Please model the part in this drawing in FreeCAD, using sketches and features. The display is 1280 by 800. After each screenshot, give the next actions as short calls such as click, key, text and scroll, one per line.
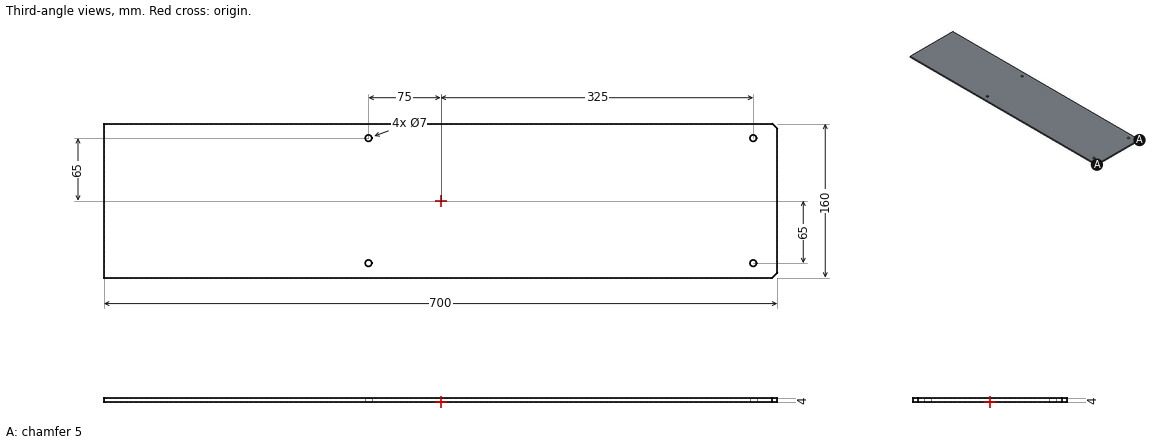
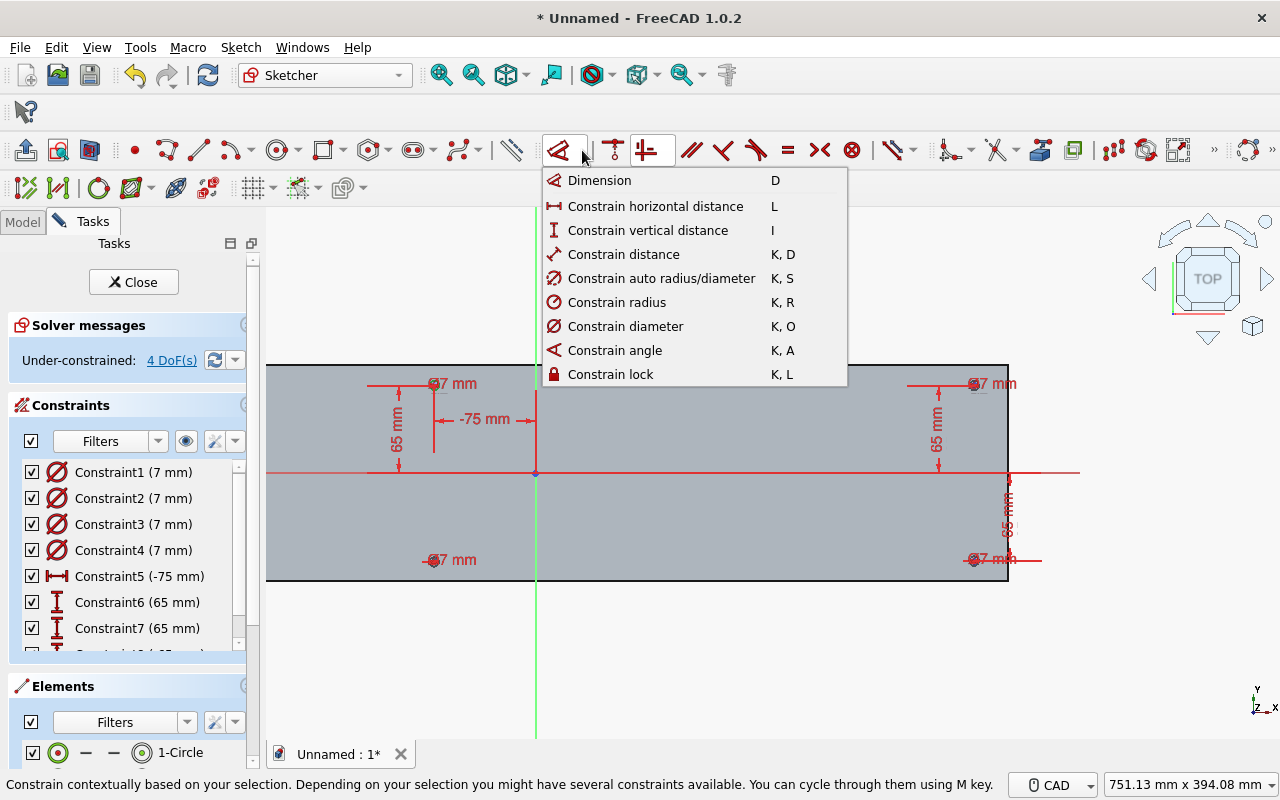
click(695, 206)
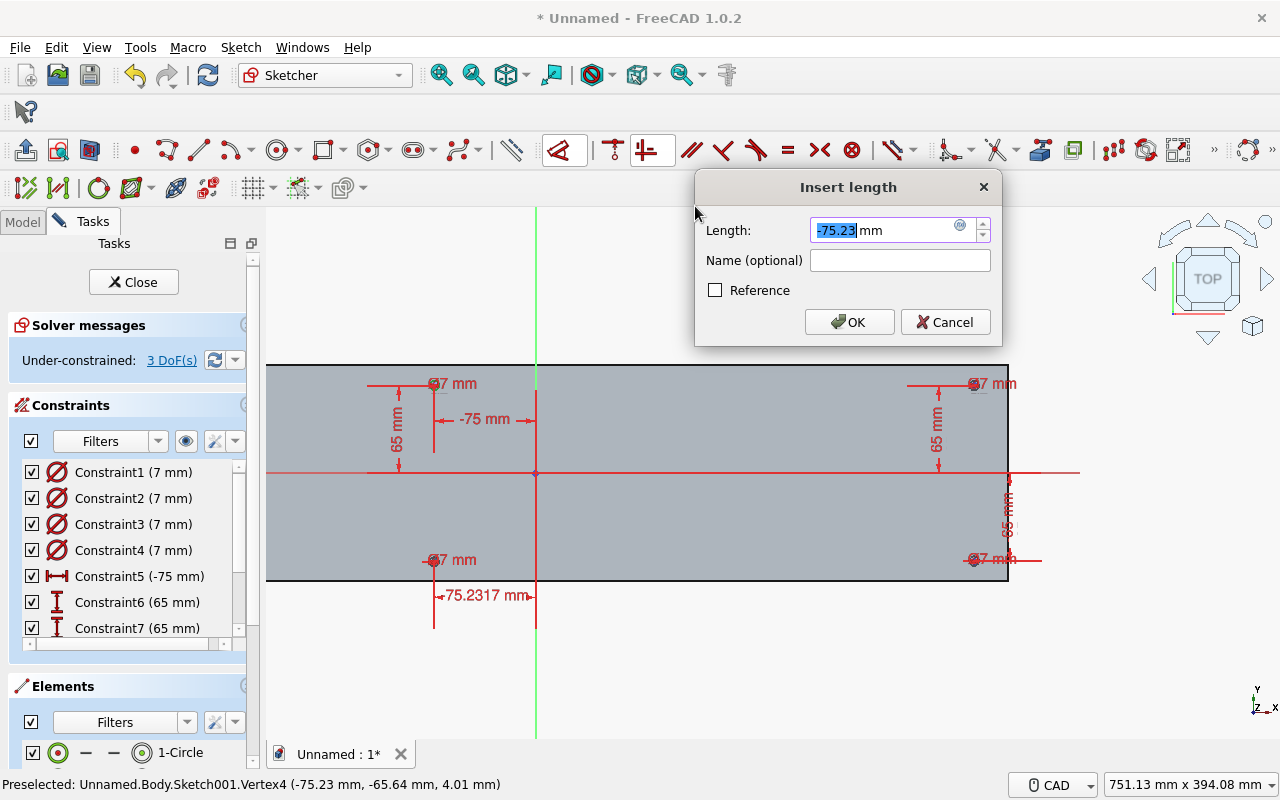
text(-75)
key(Return)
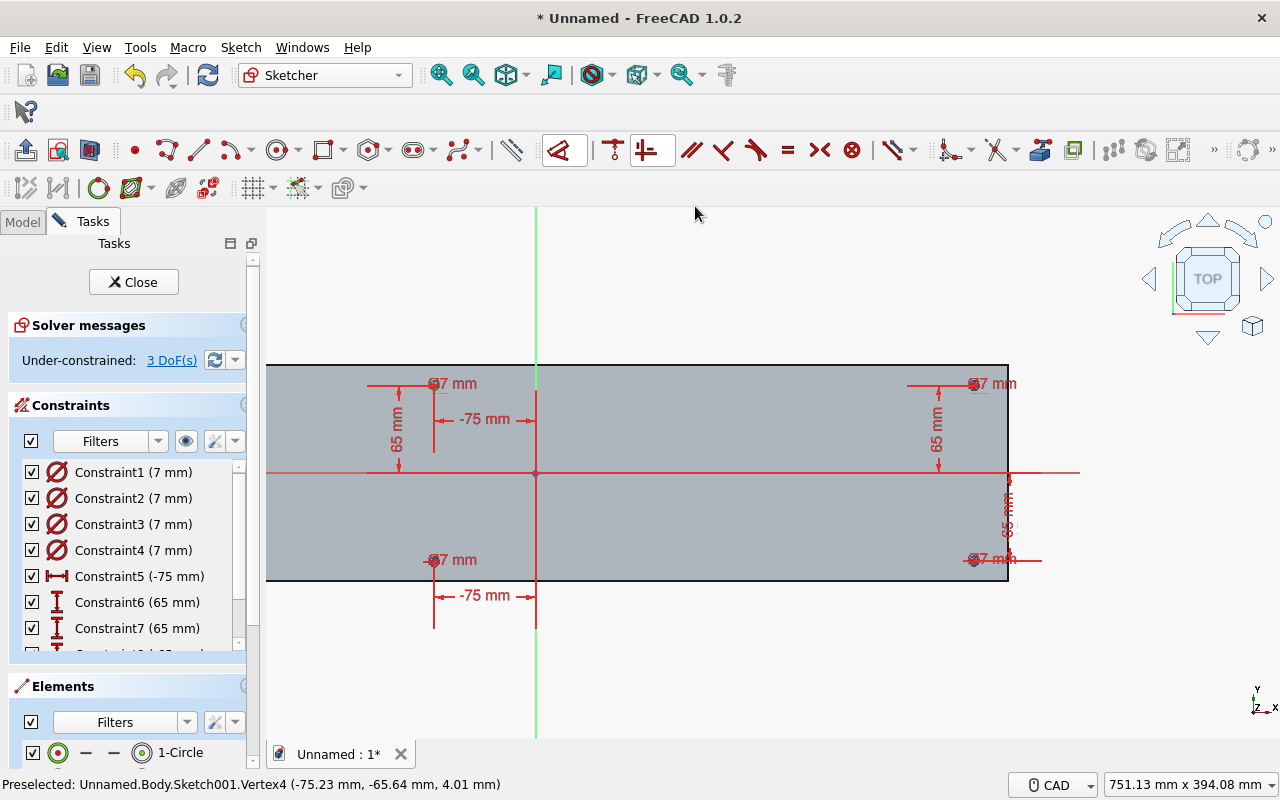
click(434, 562)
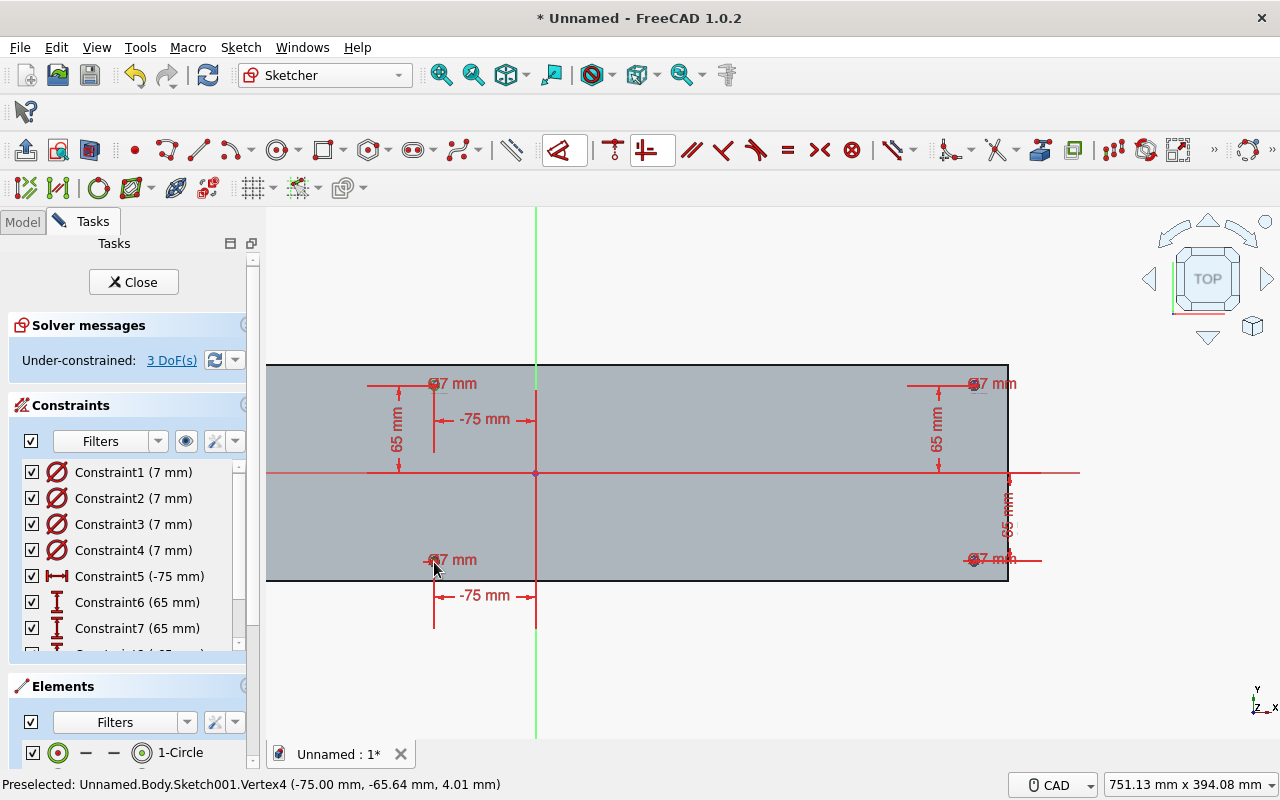
key(i)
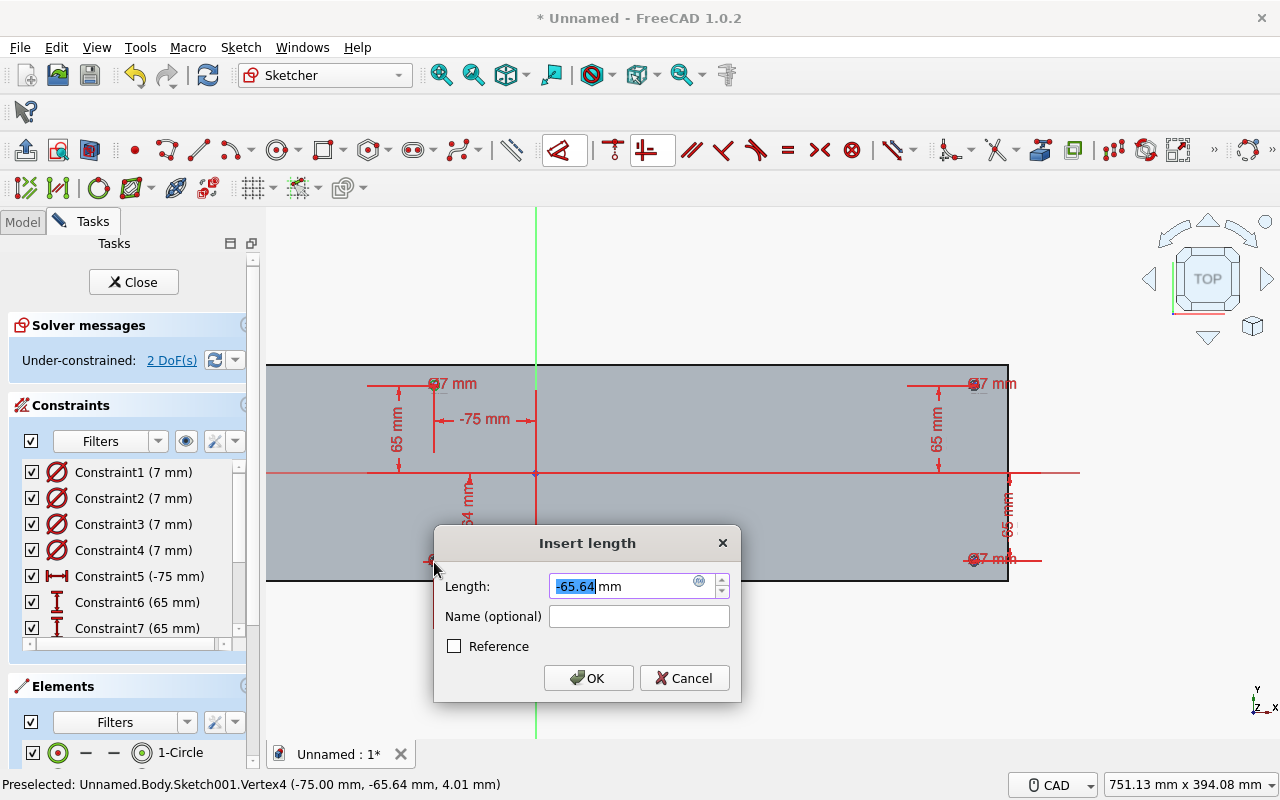
text(-65)
key(Return)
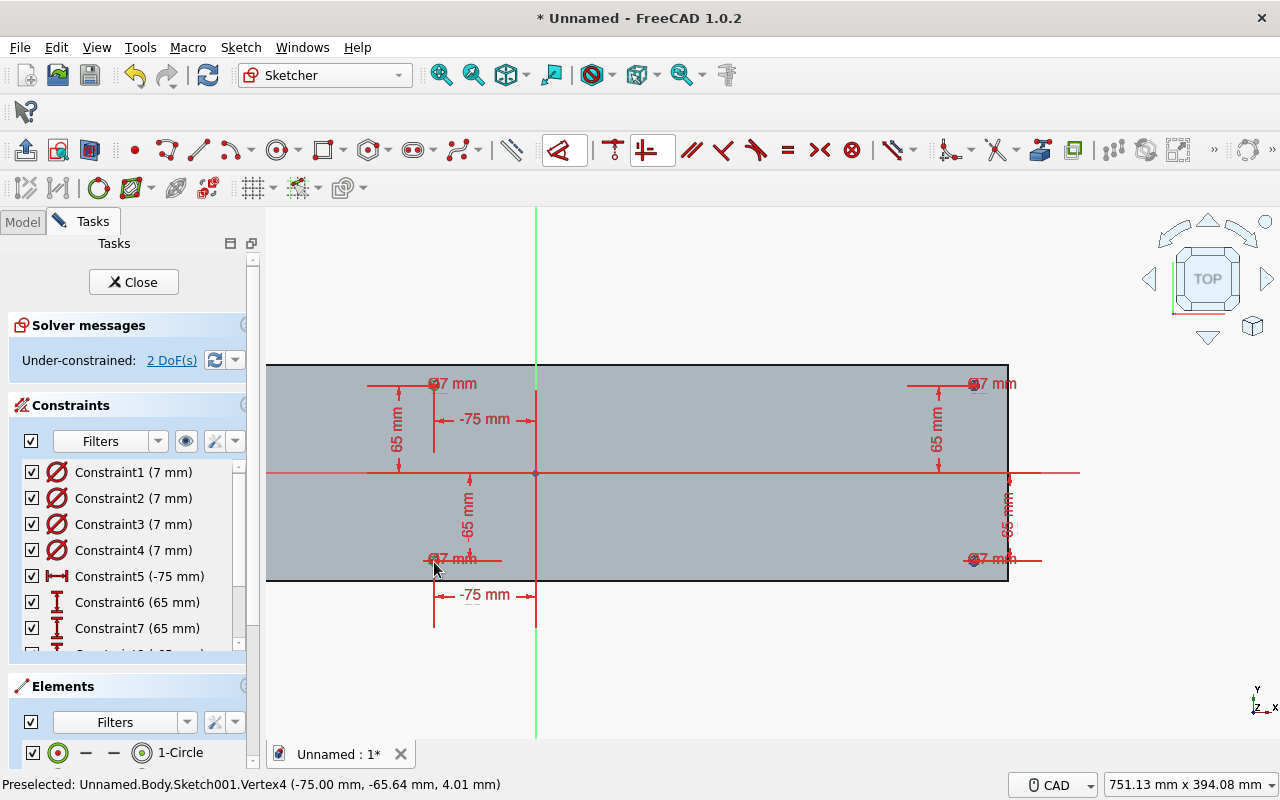
click(974, 386)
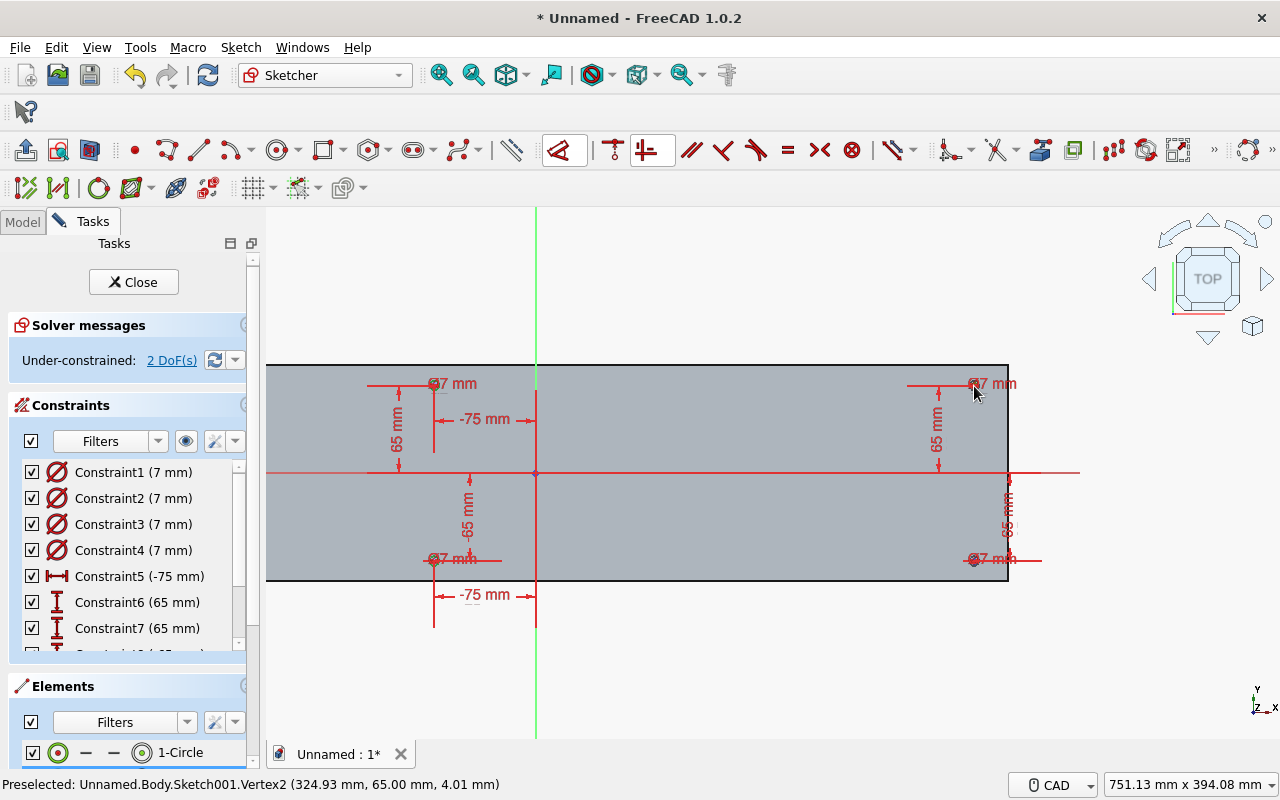
click(582, 150)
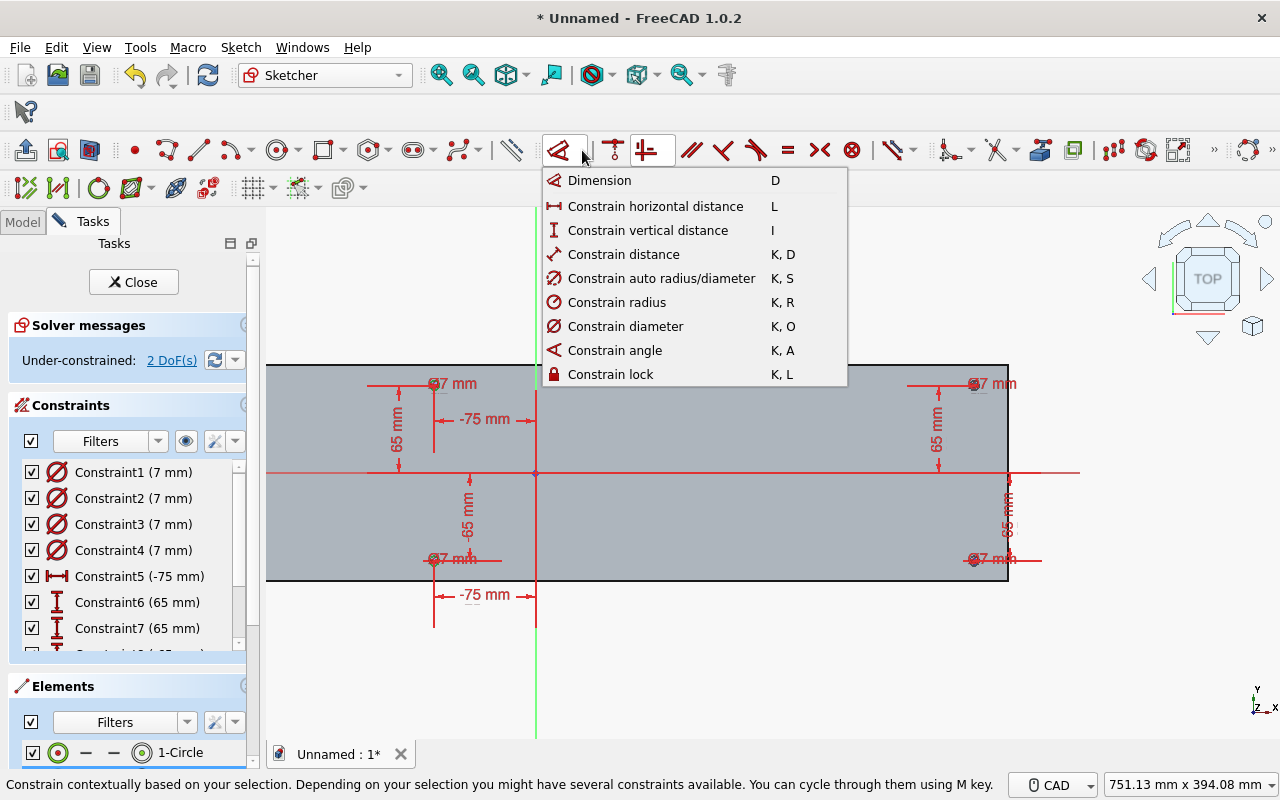
click(695, 206)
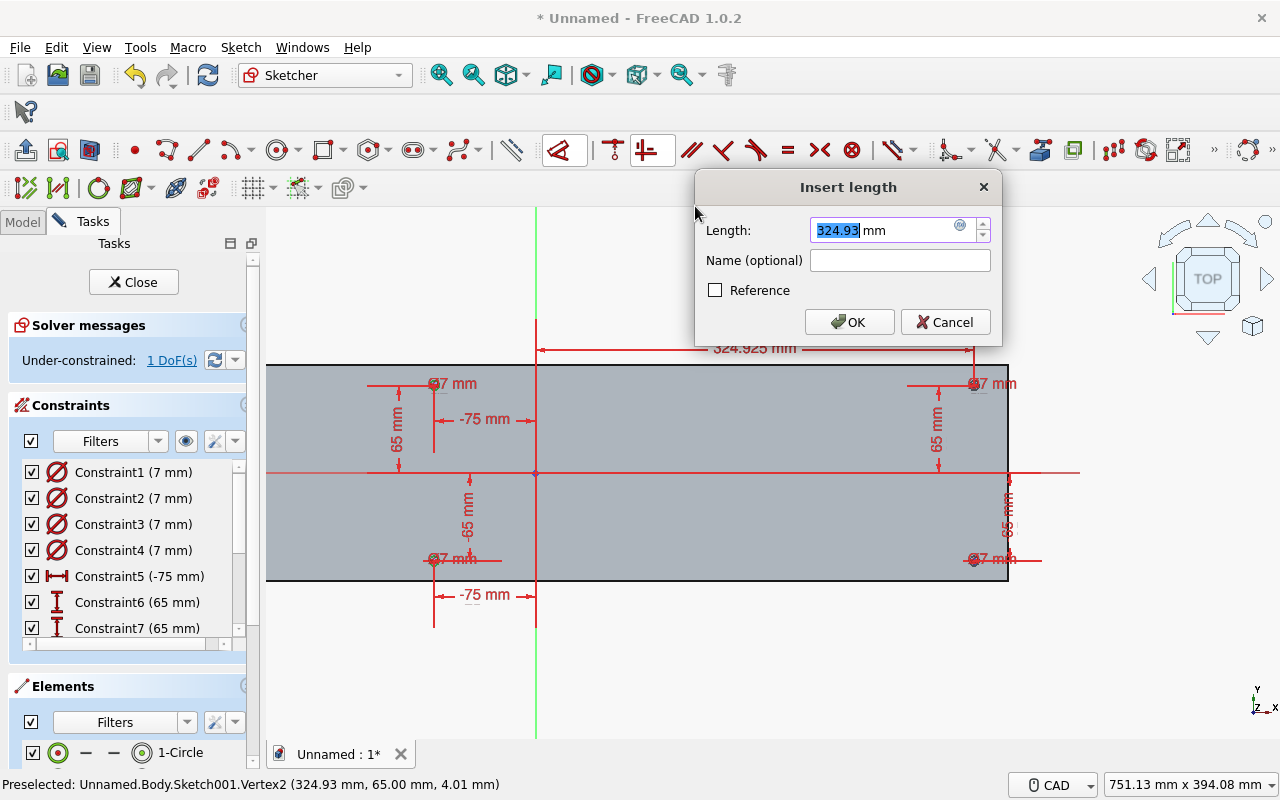
text(325)
key(Return)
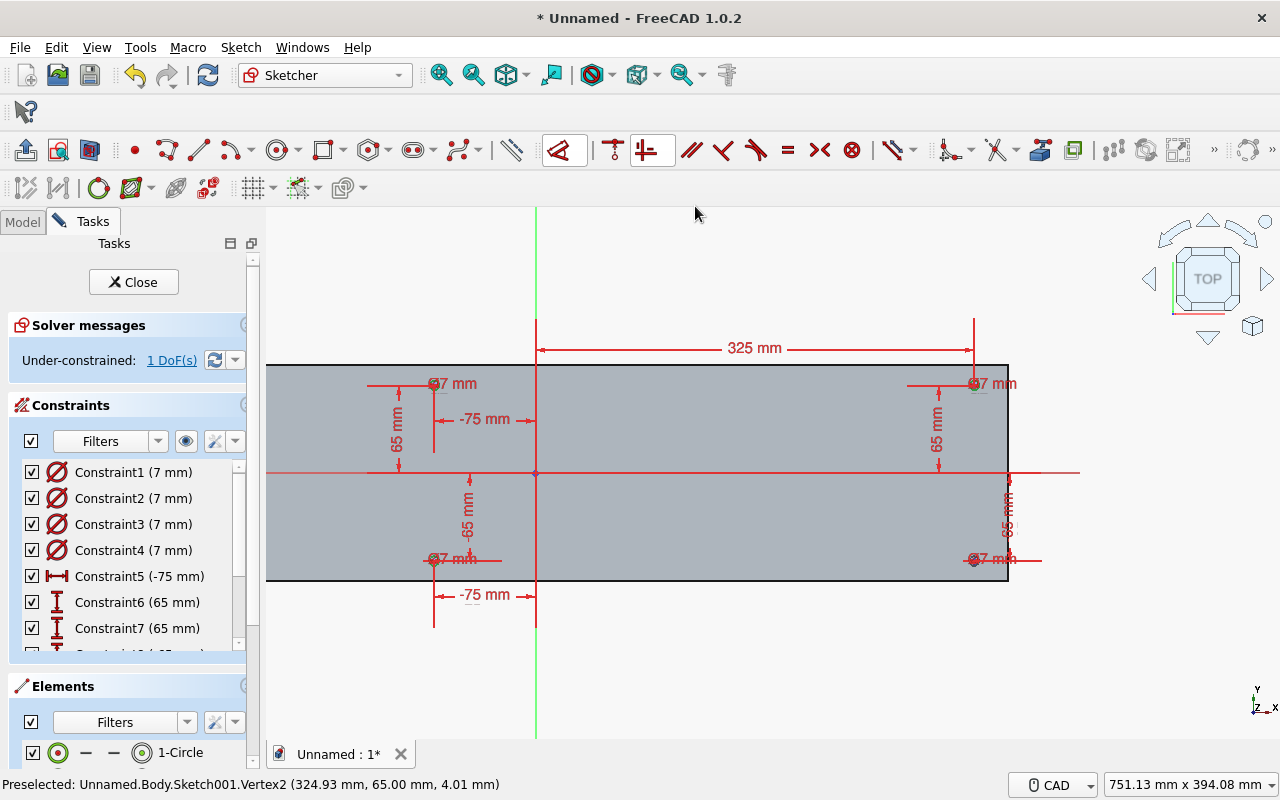
click(974, 561)